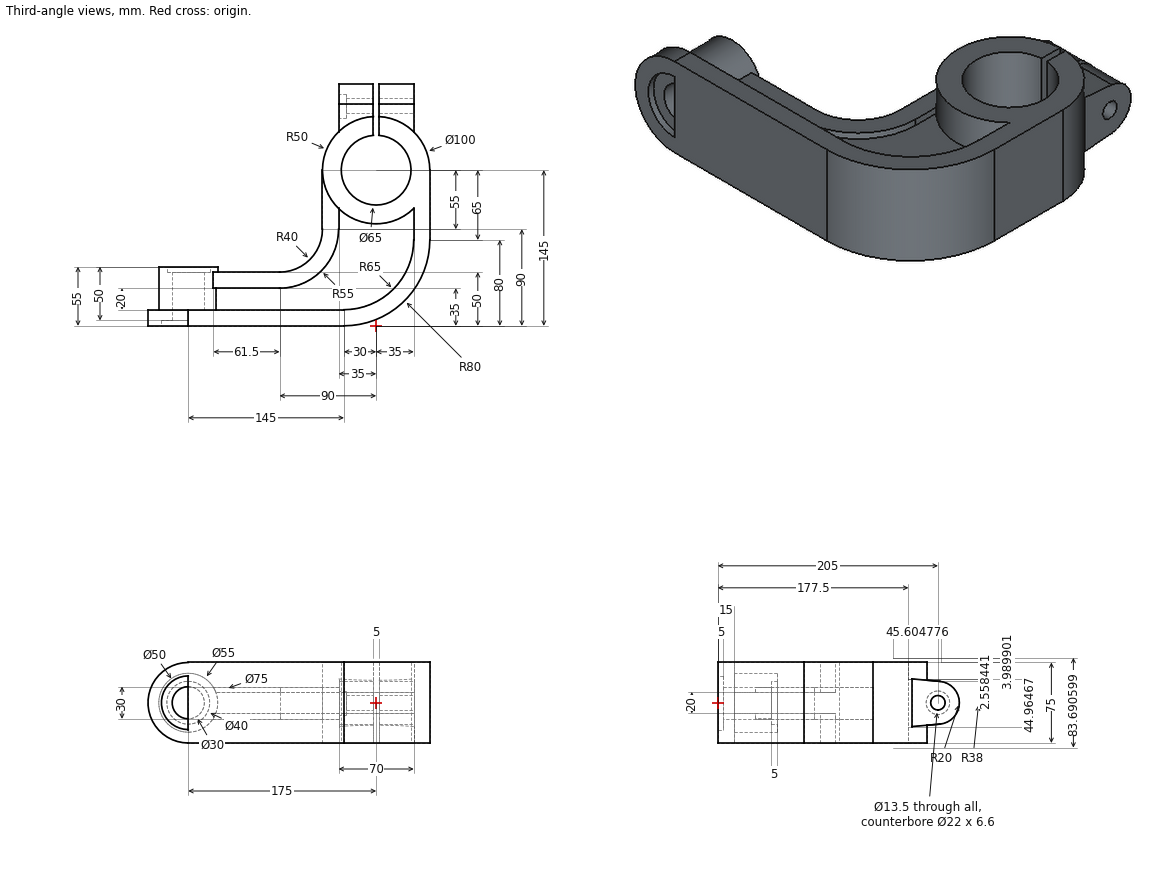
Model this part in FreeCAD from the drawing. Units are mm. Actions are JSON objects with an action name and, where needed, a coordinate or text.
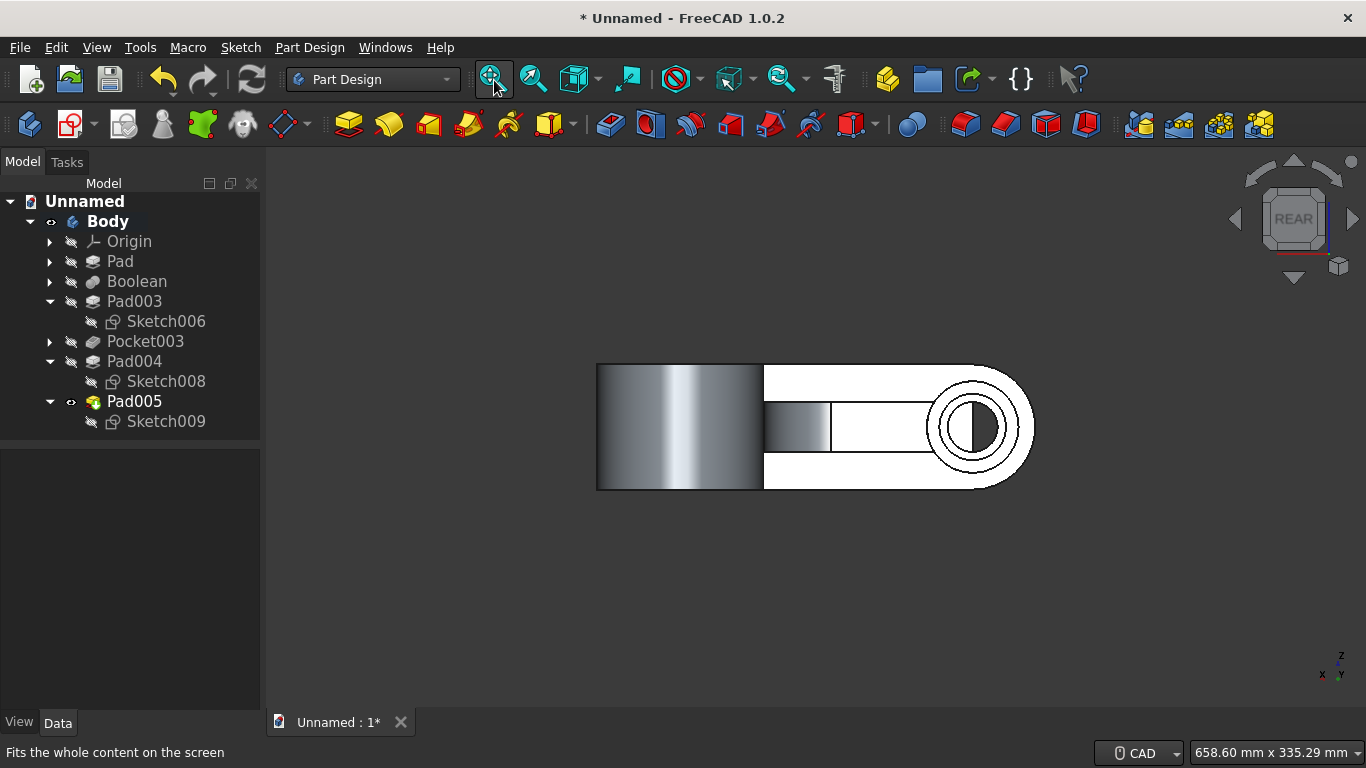
{"action": "left_click", "coordinate": [70, 124]}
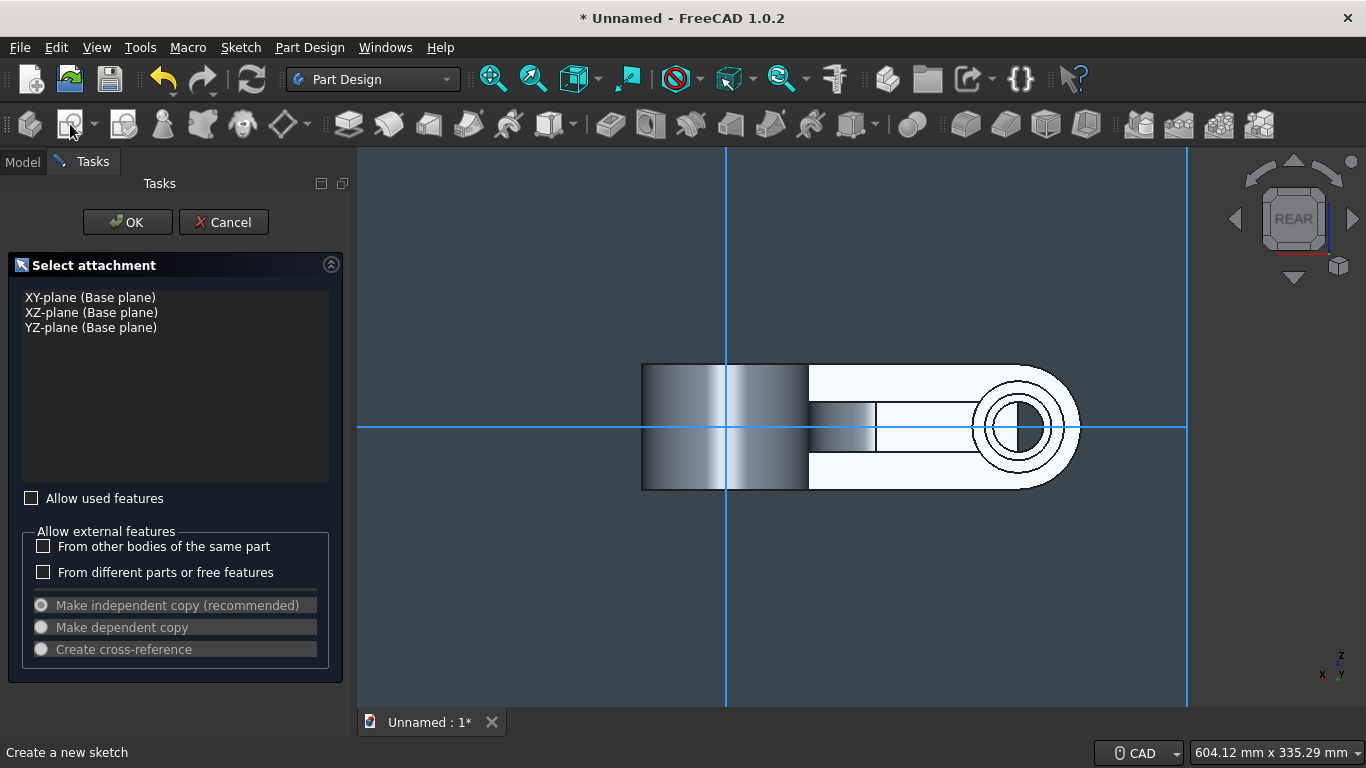
{"action": "left_click", "coordinate": [82, 328]}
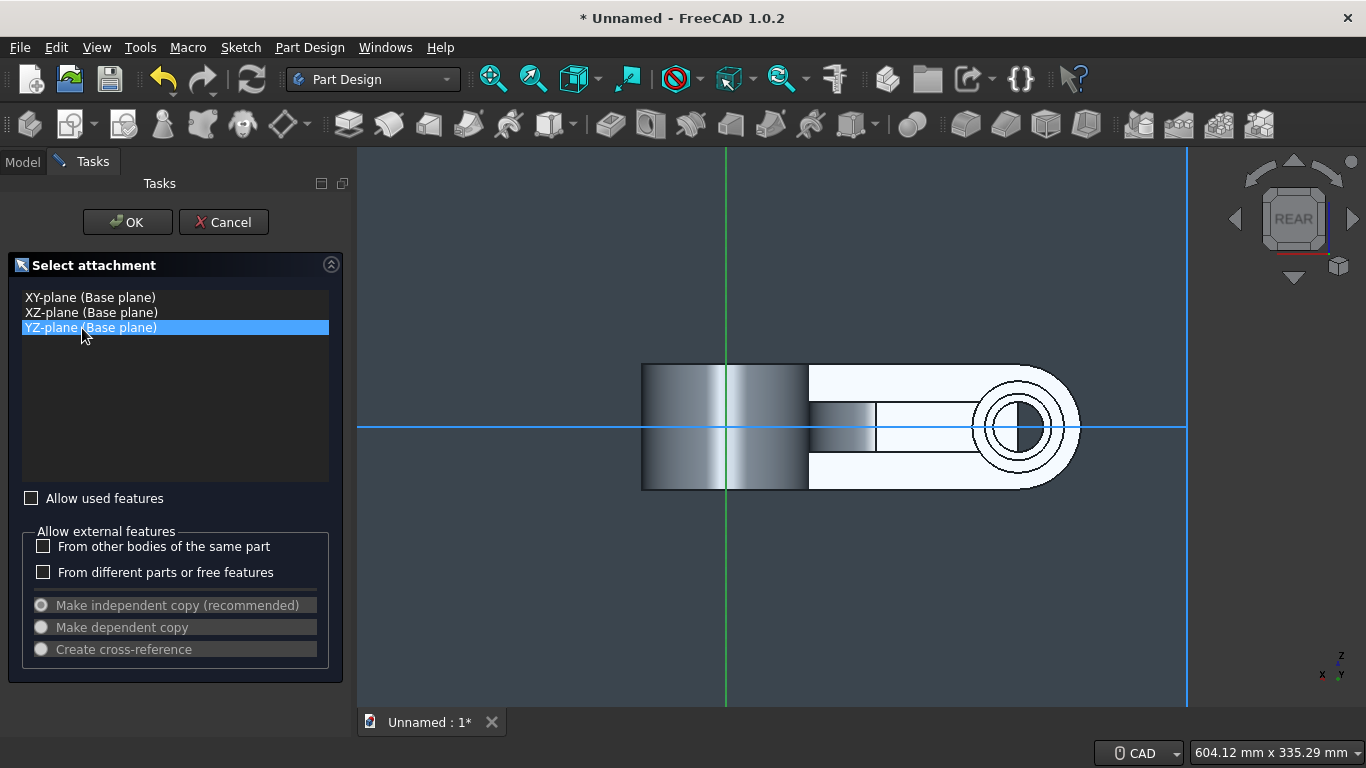
{"action": "left_click", "coordinate": [128, 222]}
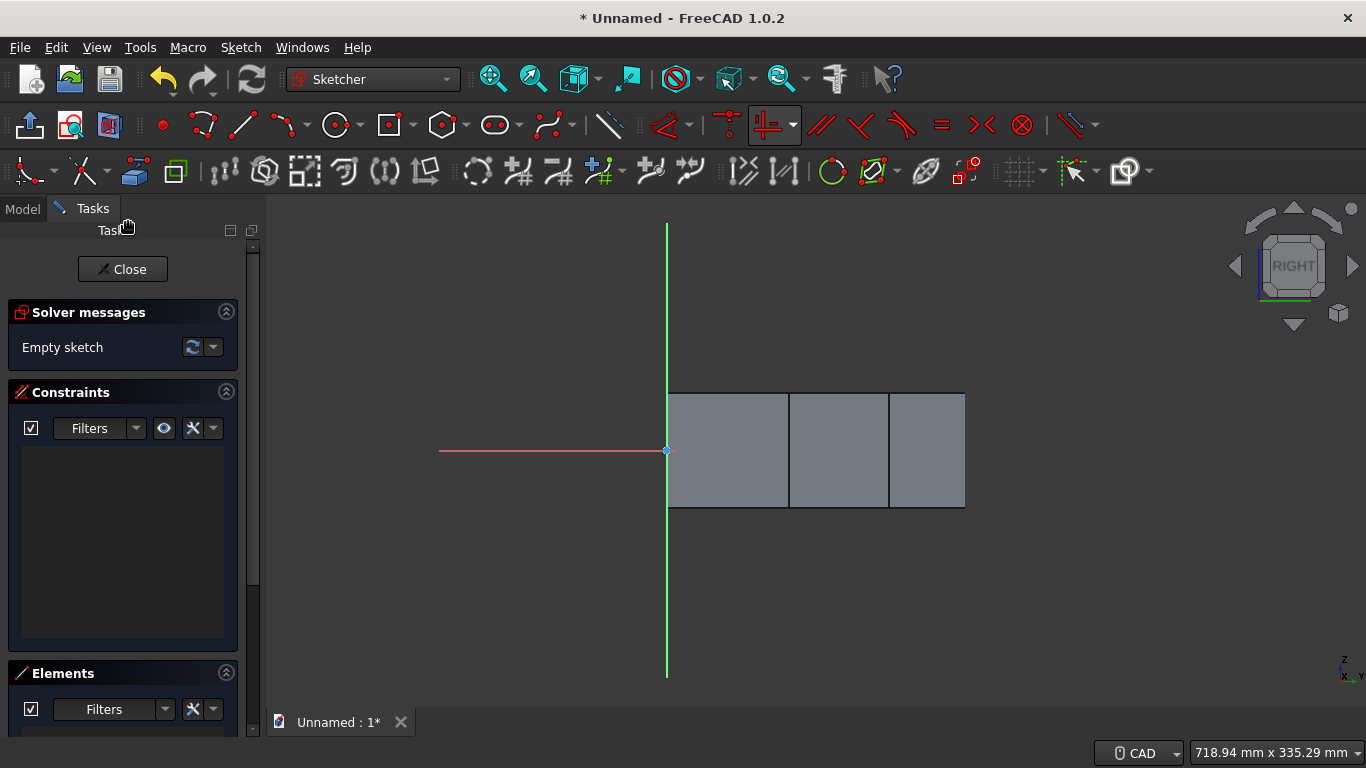
{"action": "key", "text": "q s"}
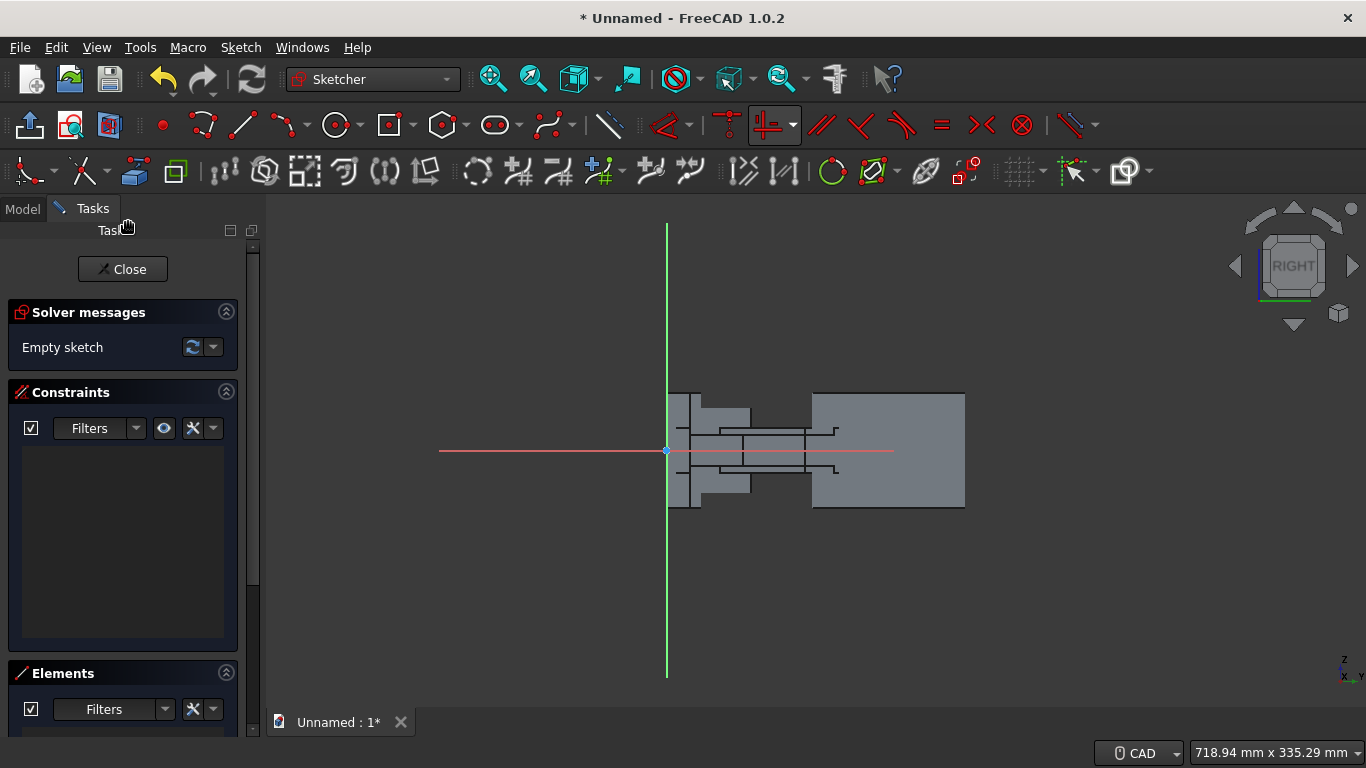
{"action": "scroll", "coordinate": [1032, 450], "scroll_direction": "up", "scroll_amount": 8}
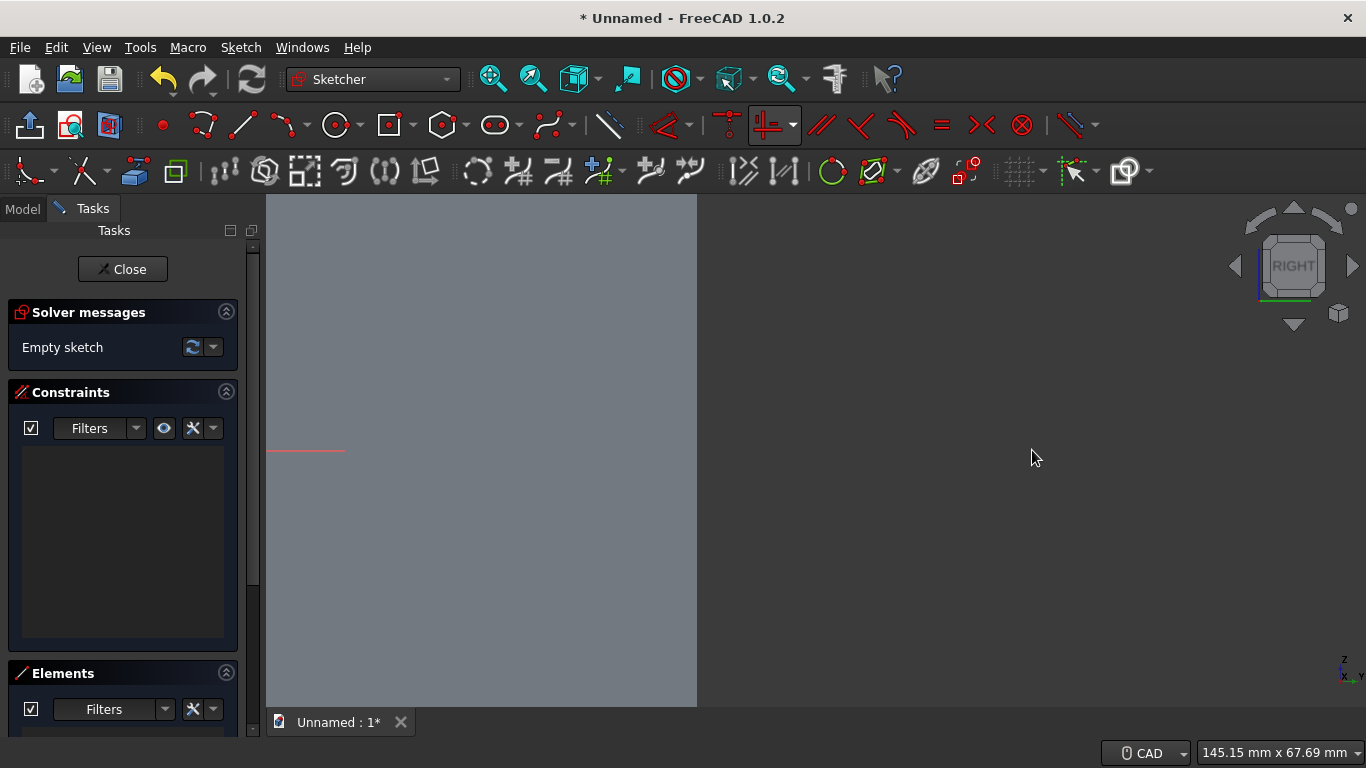
{"action": "key", "text": "g m"}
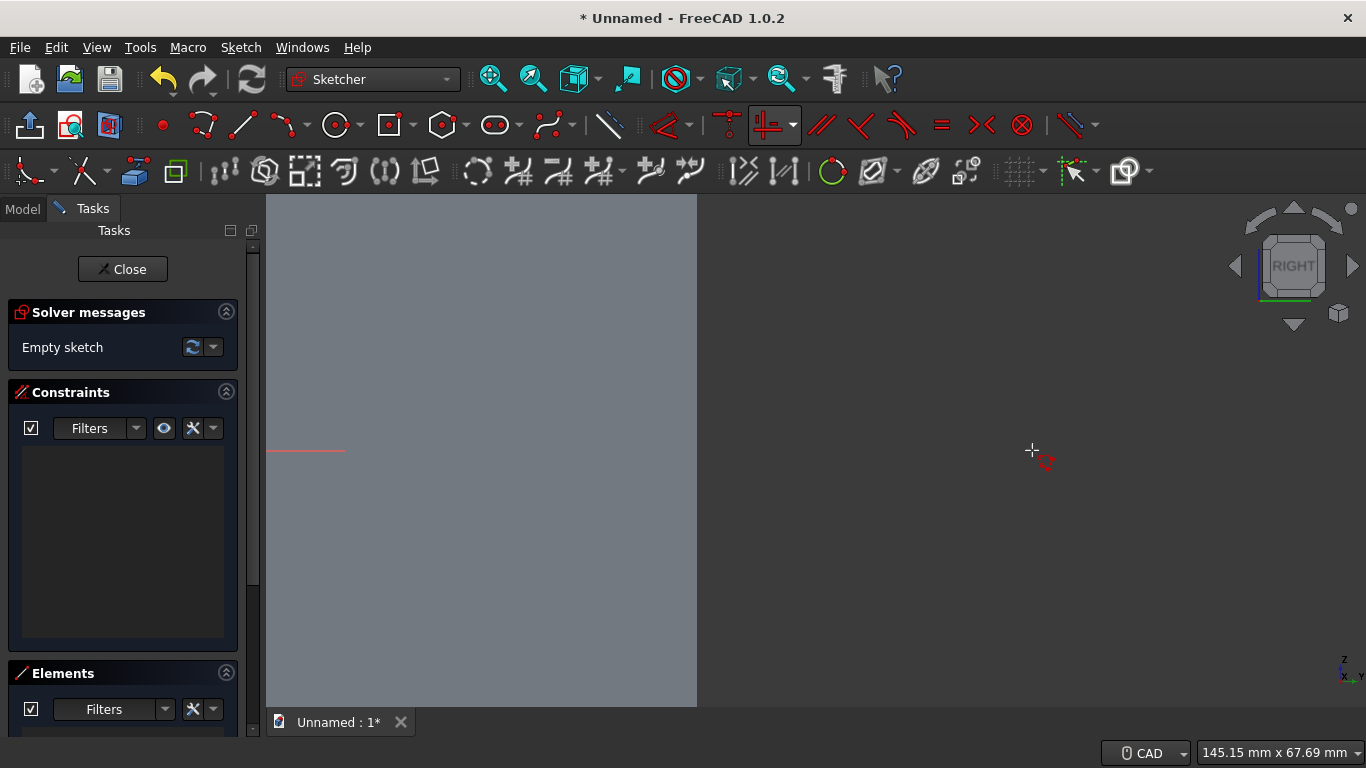
{"action": "left_click", "coordinate": [788, 300]}
{"action": "left_click", "coordinate": [566, 280]}
{"action": "left_click", "coordinate": [566, 621]}
{"action": "left_click", "coordinate": [788, 601]}
{"action": "right_click", "coordinate": [788, 601]}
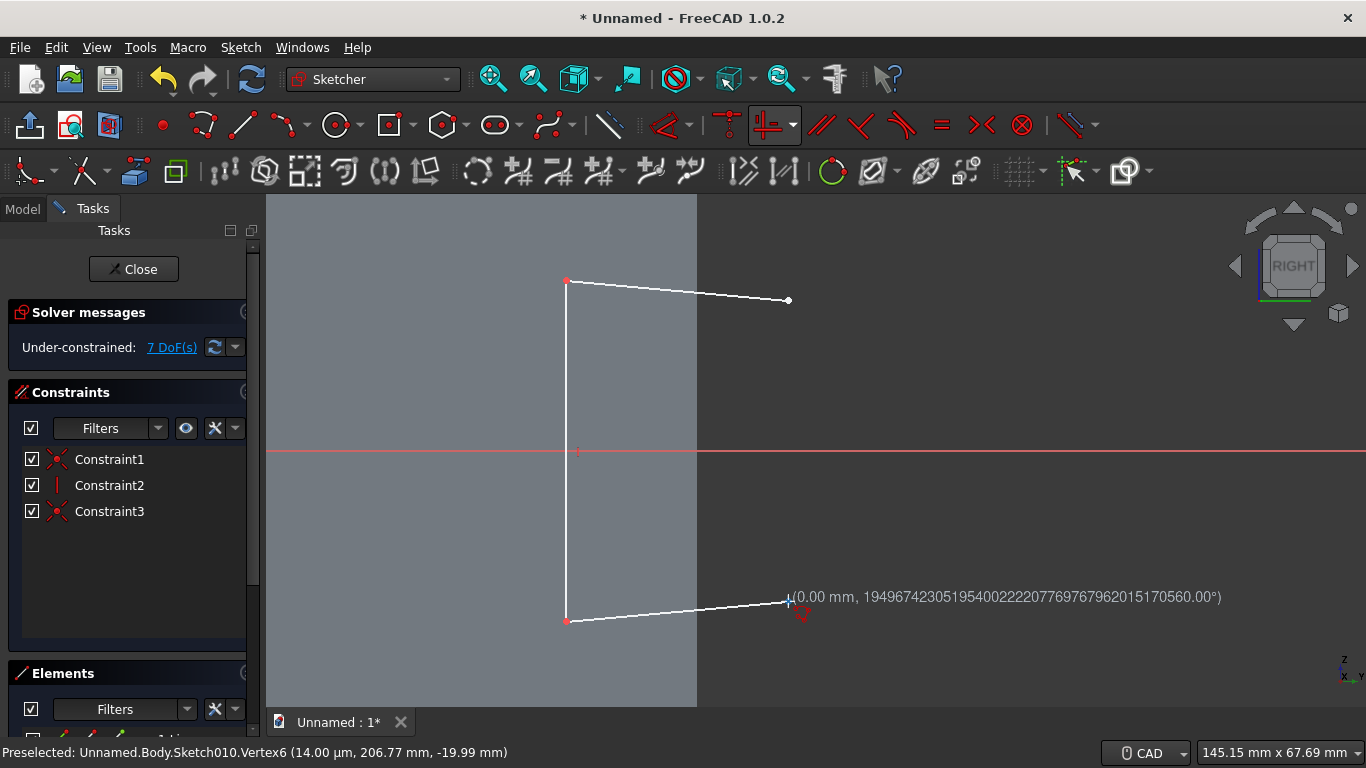
{"action": "key", "text": "g 3 a"}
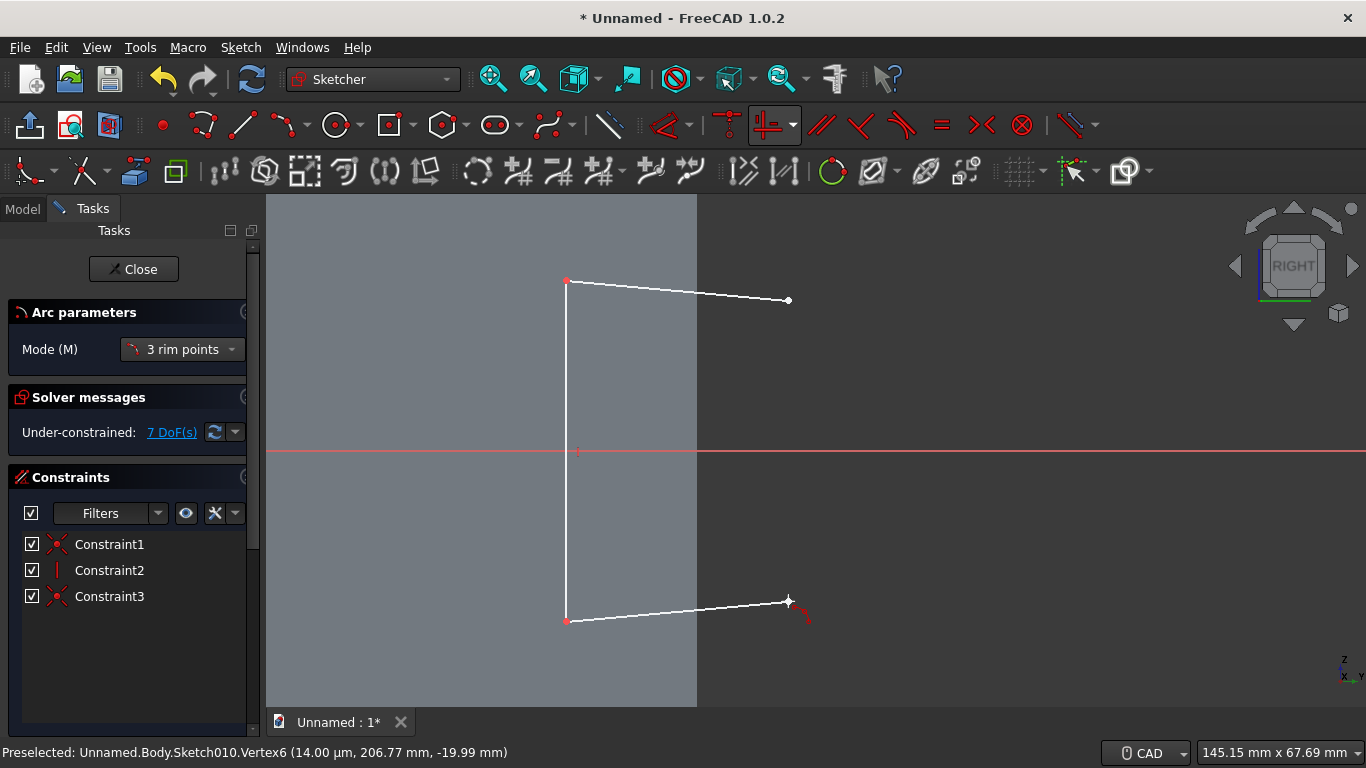
{"action": "left_click", "coordinate": [788, 602]}
{"action": "left_click", "coordinate": [788, 301]}
{"action": "left_click", "coordinate": [920, 495]}
{"action": "key", "text": "Escape"}